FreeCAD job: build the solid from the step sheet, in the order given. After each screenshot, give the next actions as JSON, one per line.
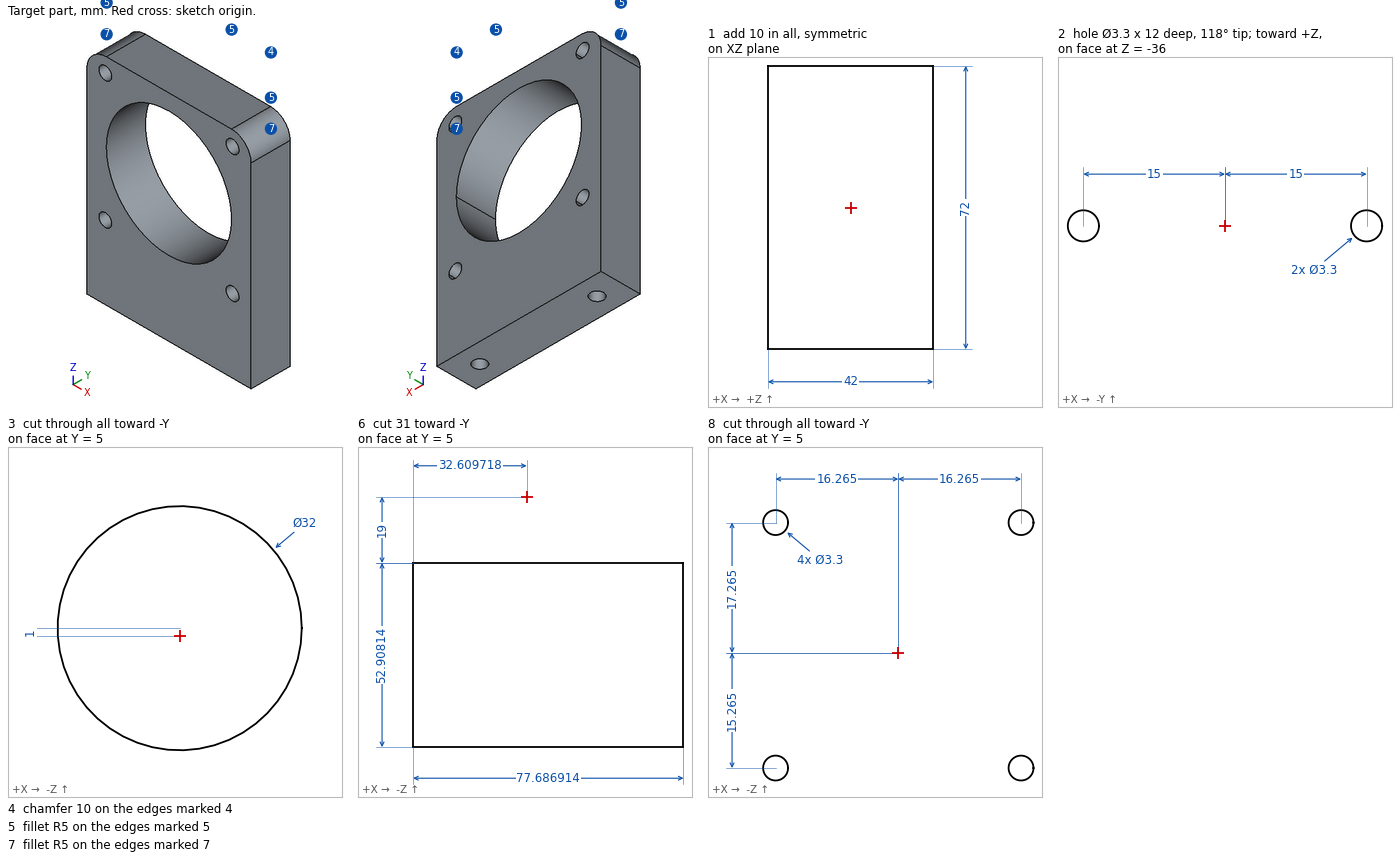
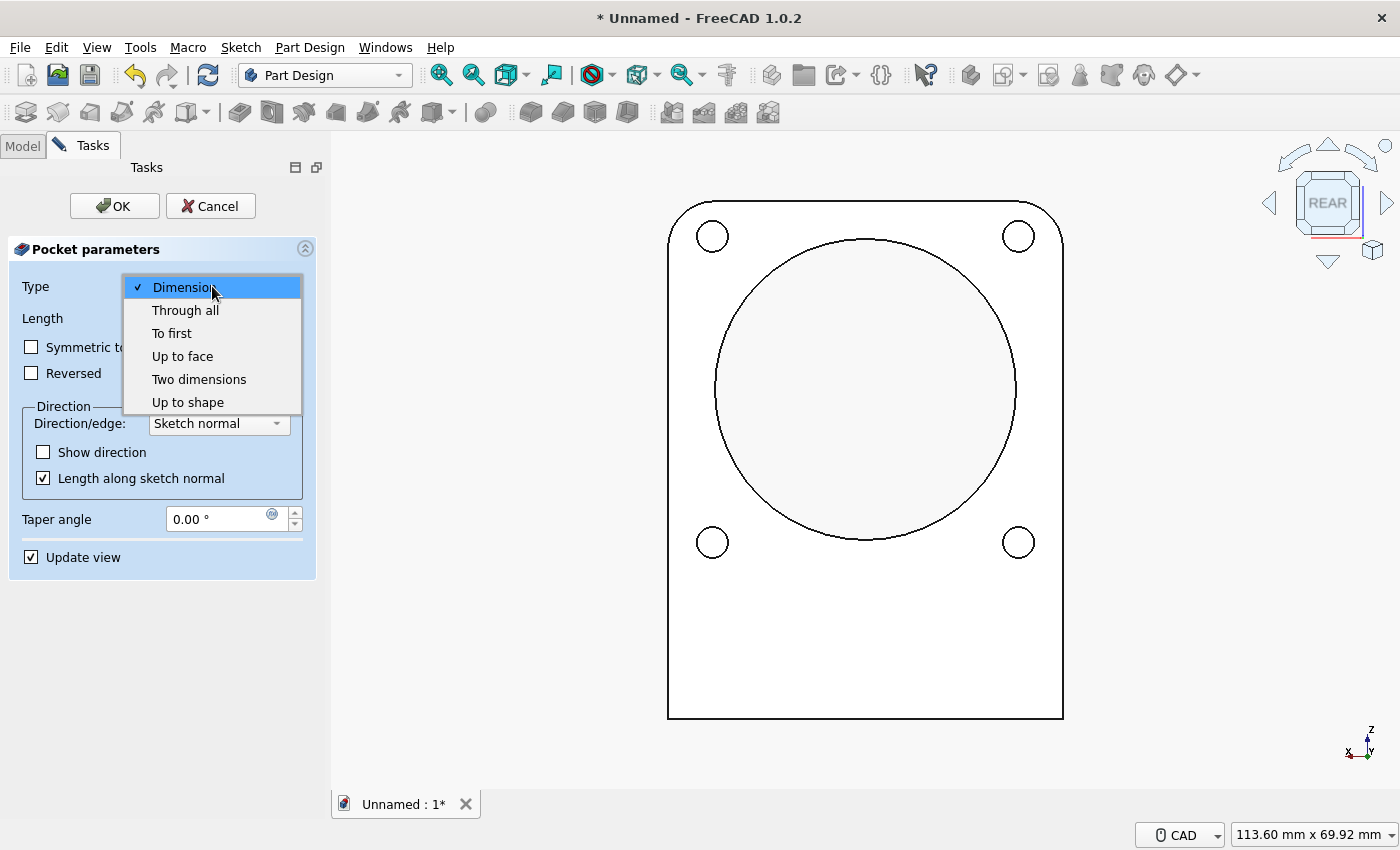
{"action": "left_click", "coordinate": [212, 310]}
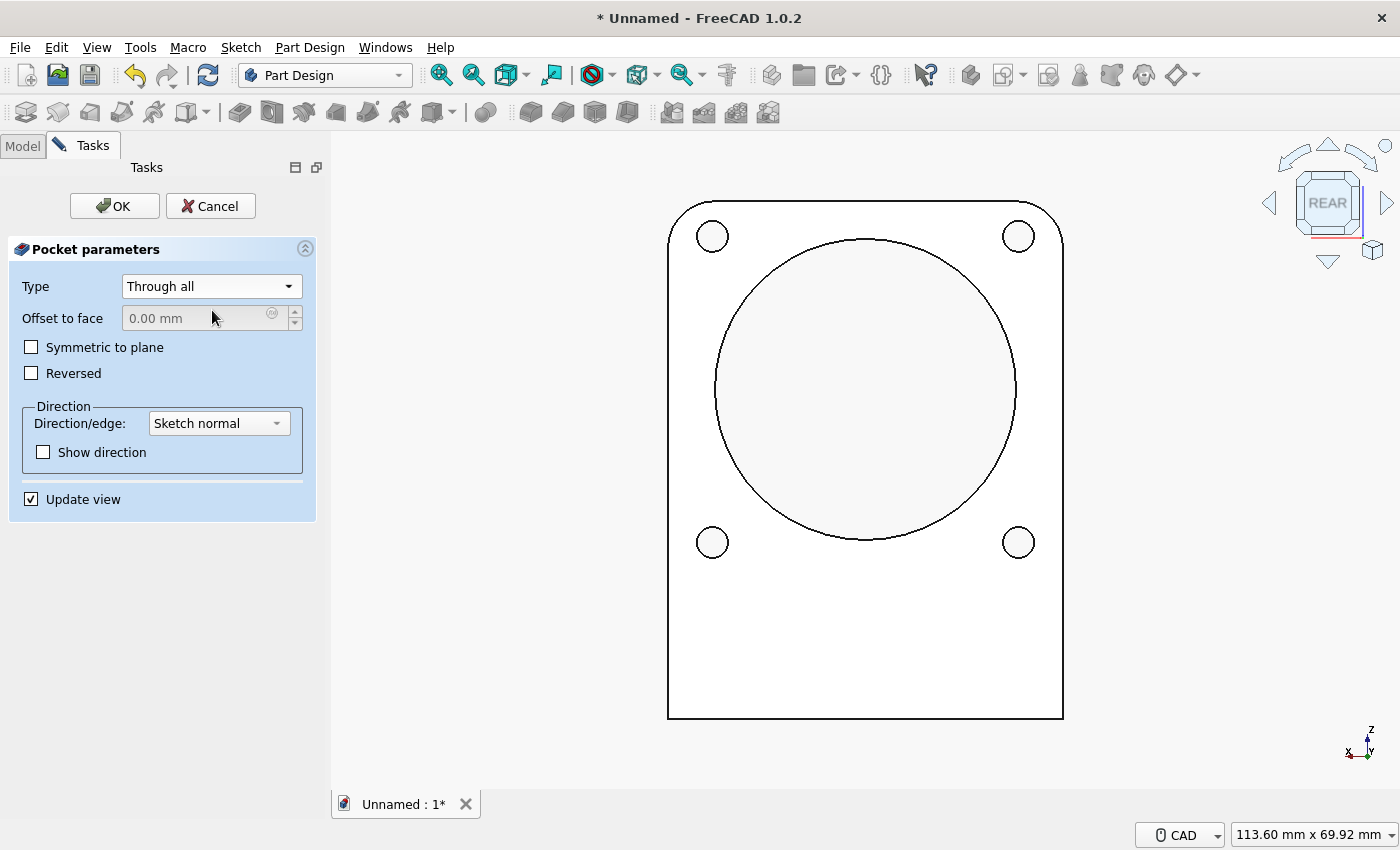
{"action": "left_click", "coordinate": [115, 206]}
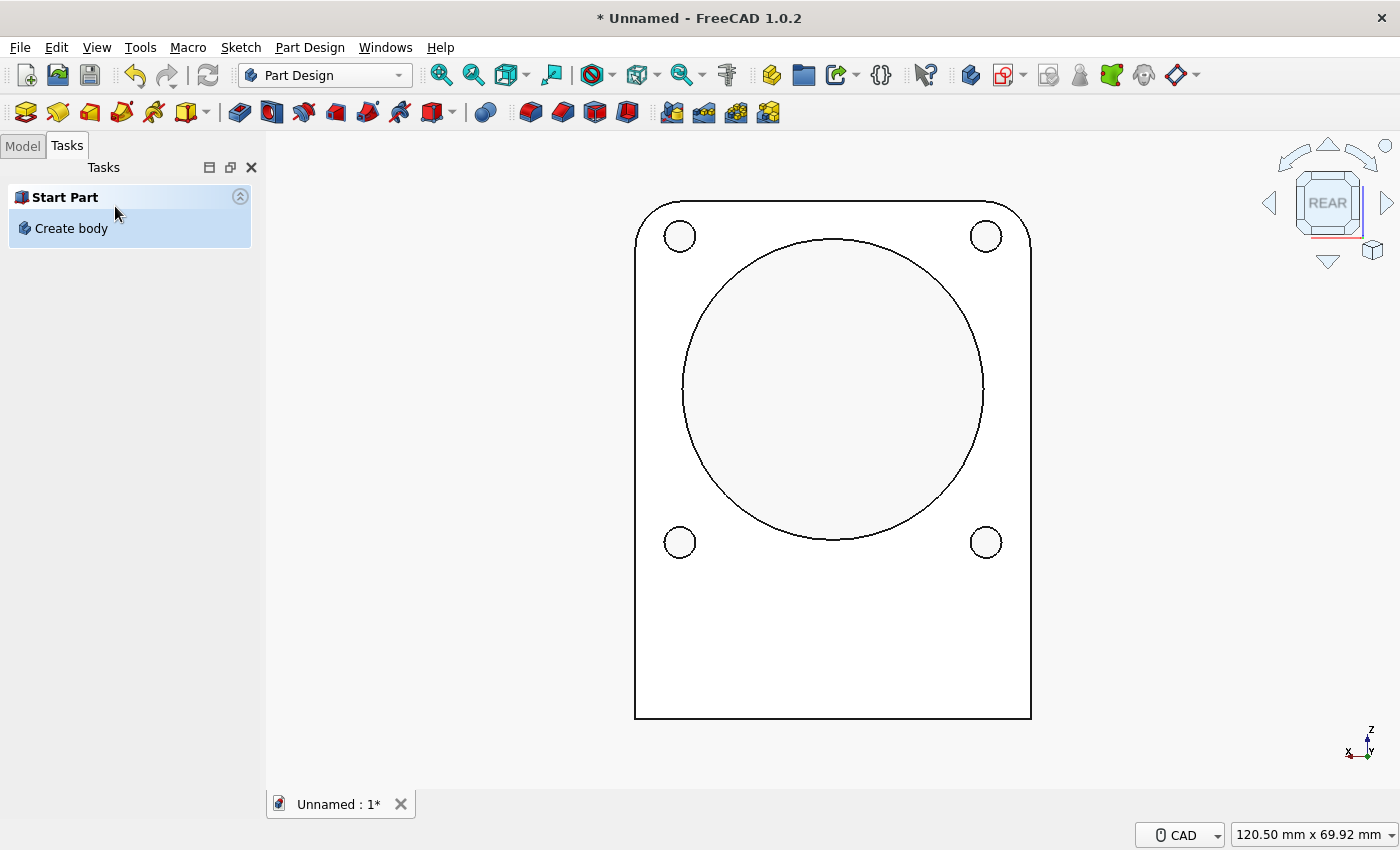
{"action": "key", "text": "0"}